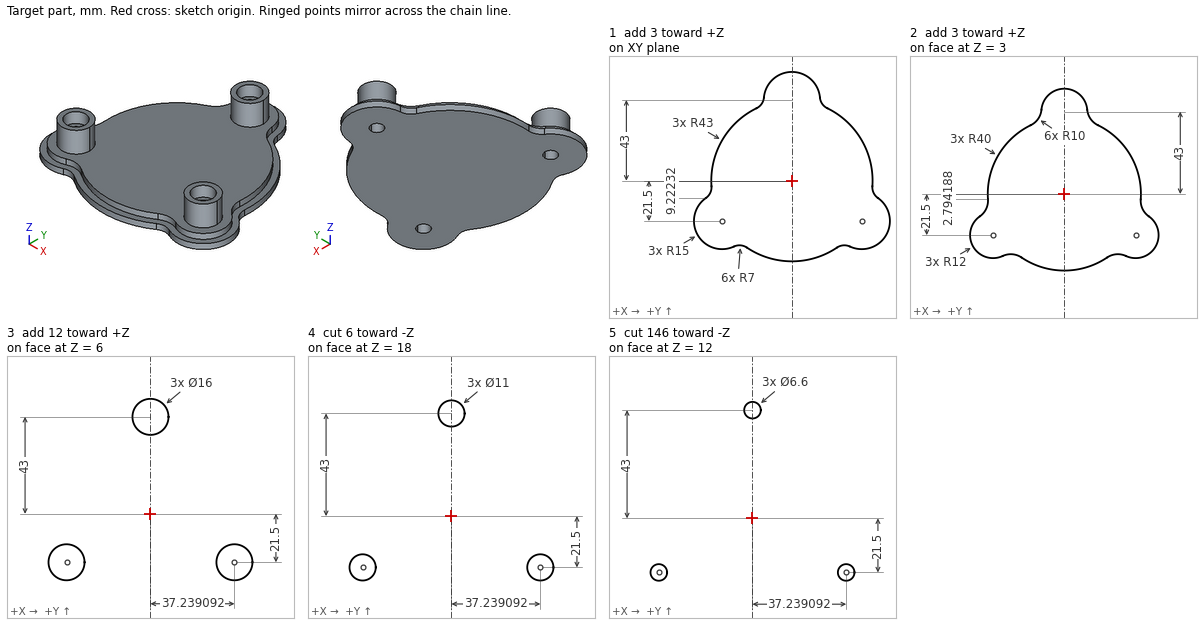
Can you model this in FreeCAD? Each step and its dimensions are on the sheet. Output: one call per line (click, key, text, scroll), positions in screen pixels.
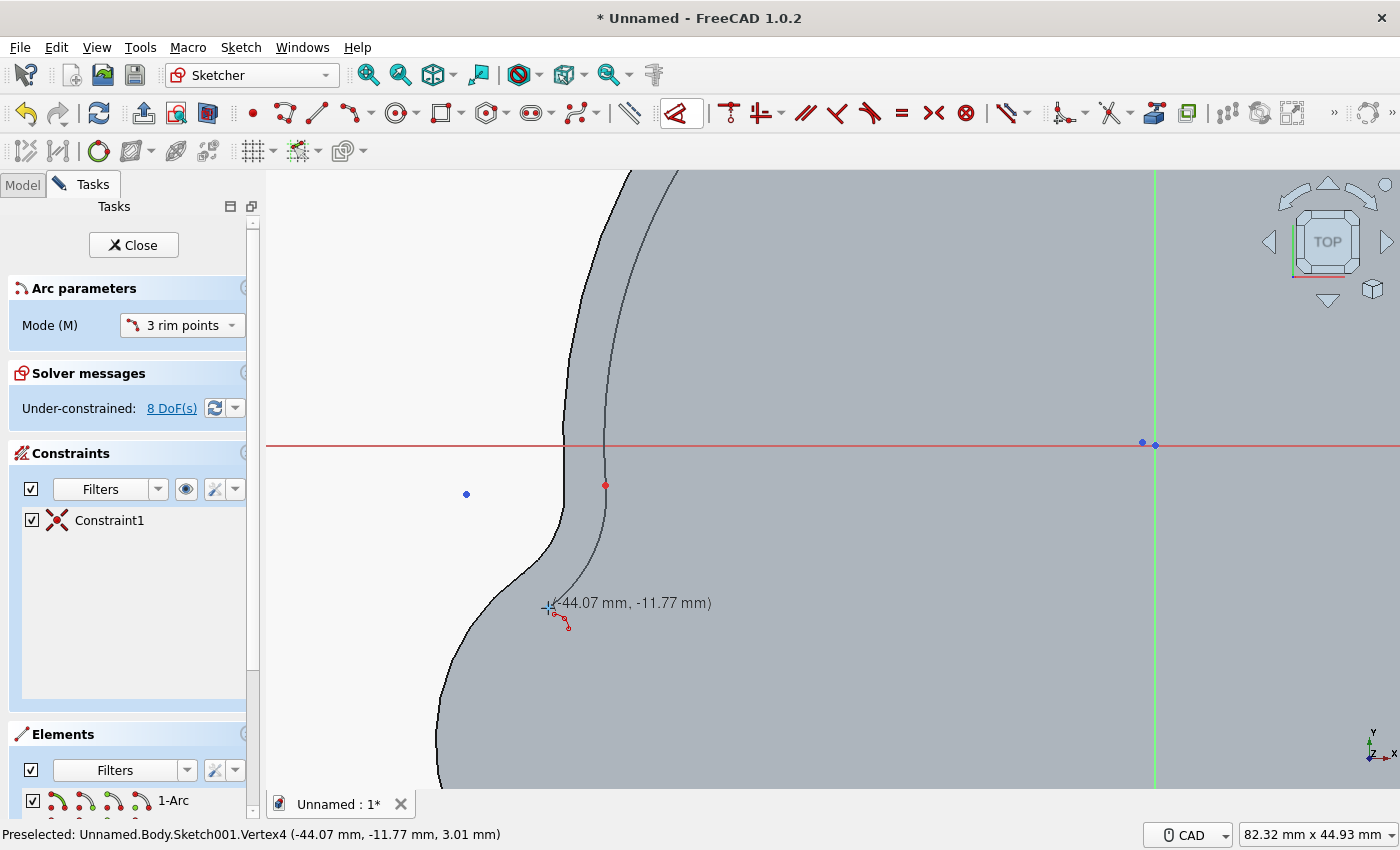
scroll(596, 539, down, 6)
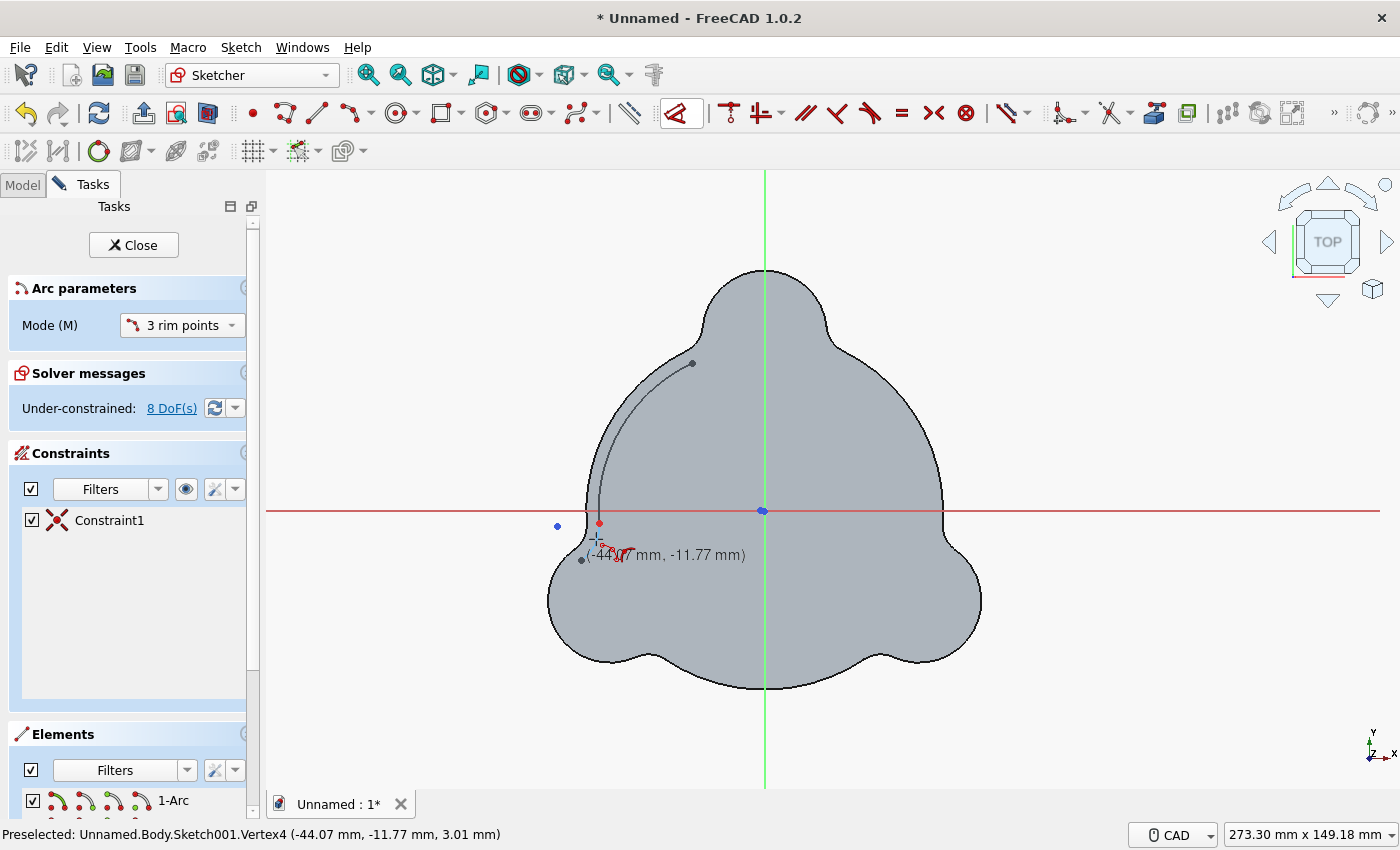
click(631, 646)
click(567, 625)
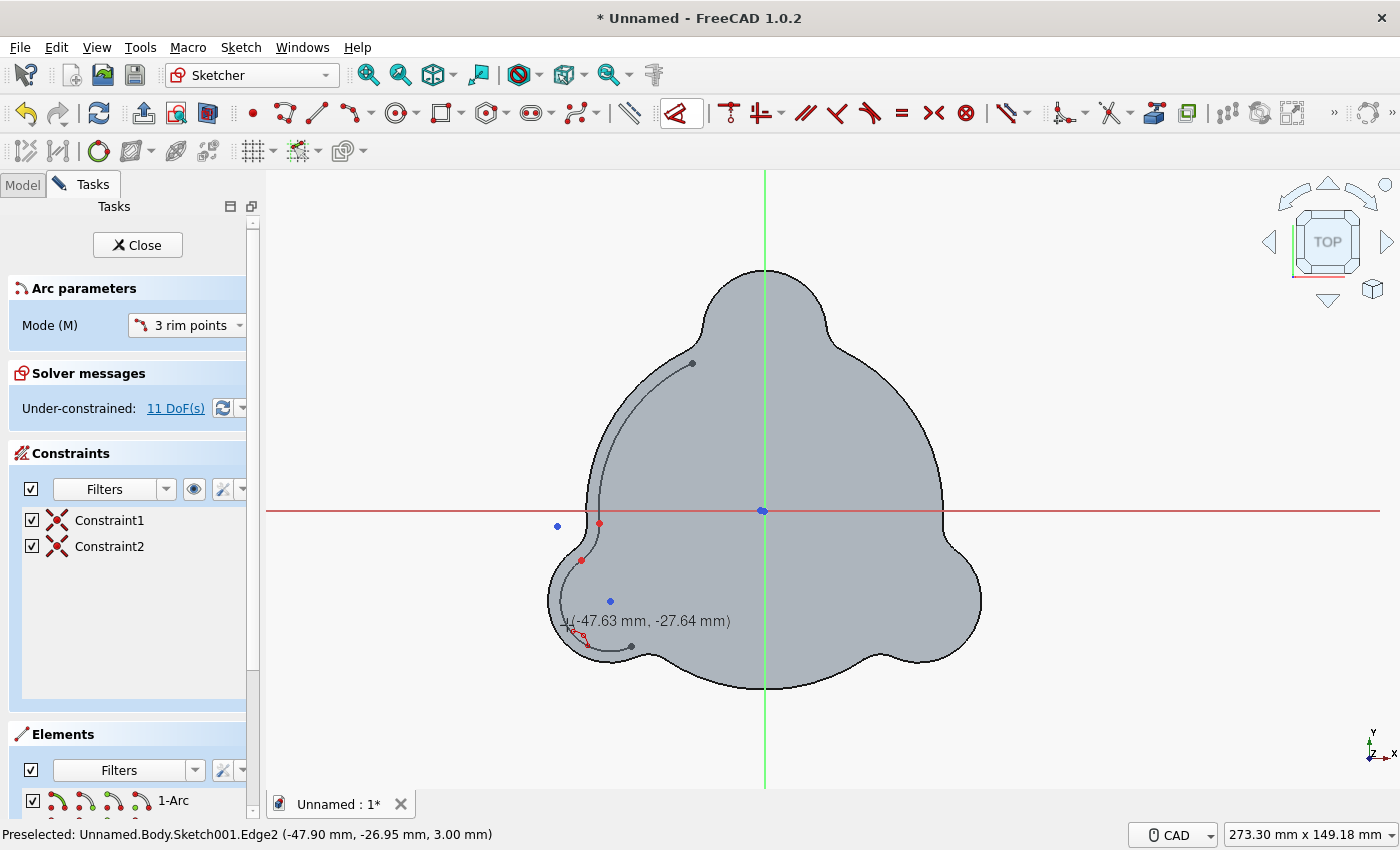
click(631, 647)
click(672, 649)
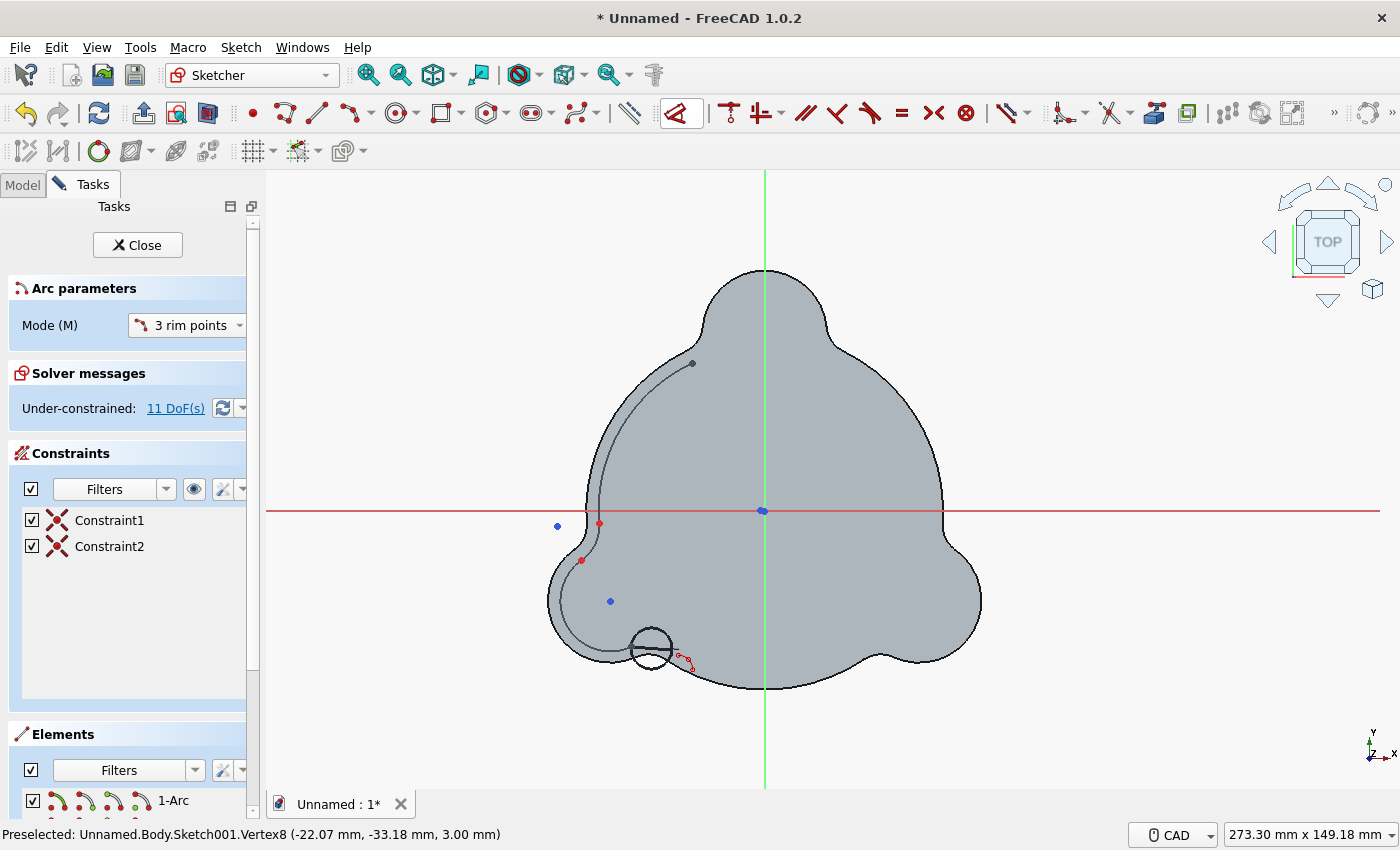
scroll(652, 642, up, 6)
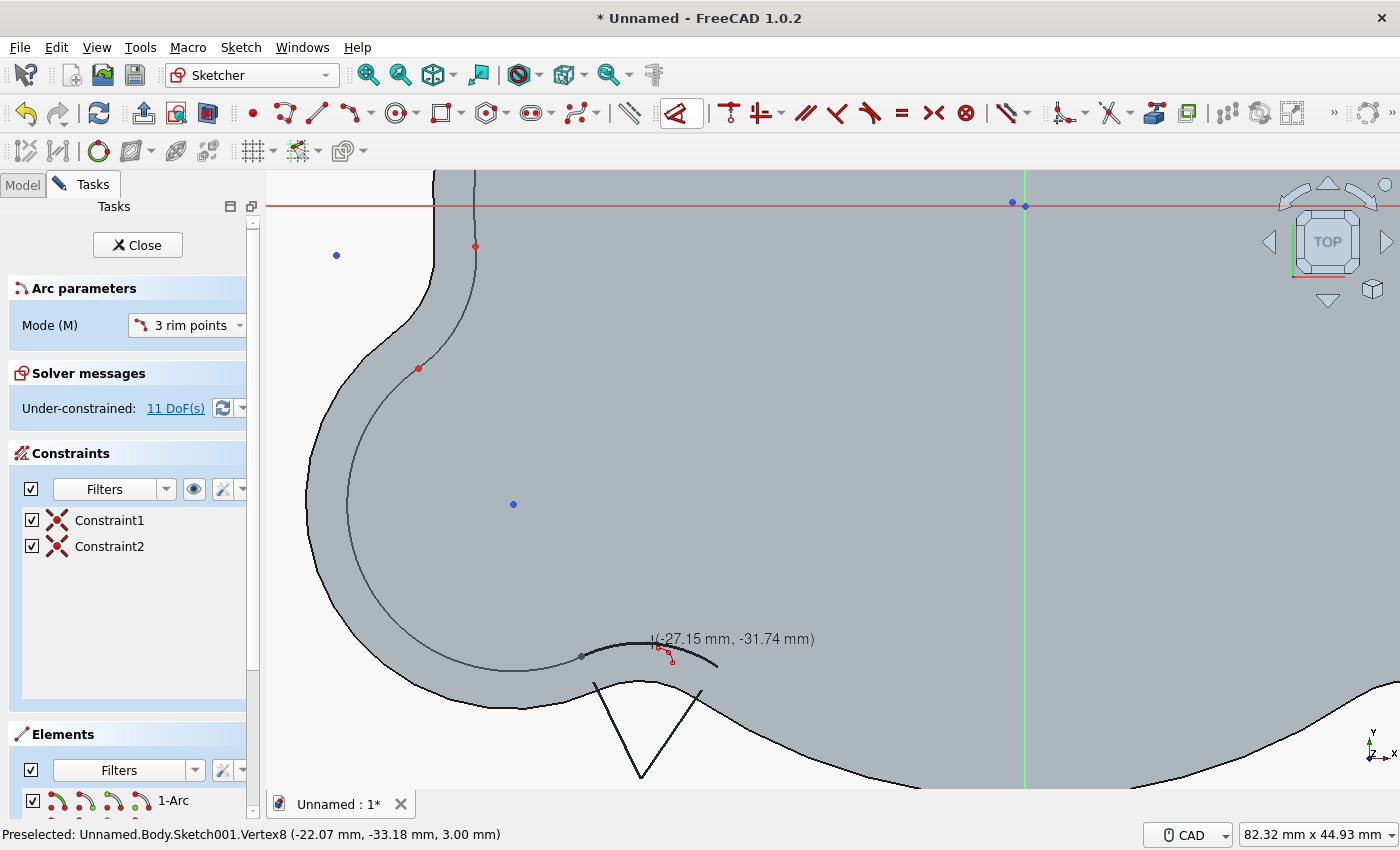
click(651, 640)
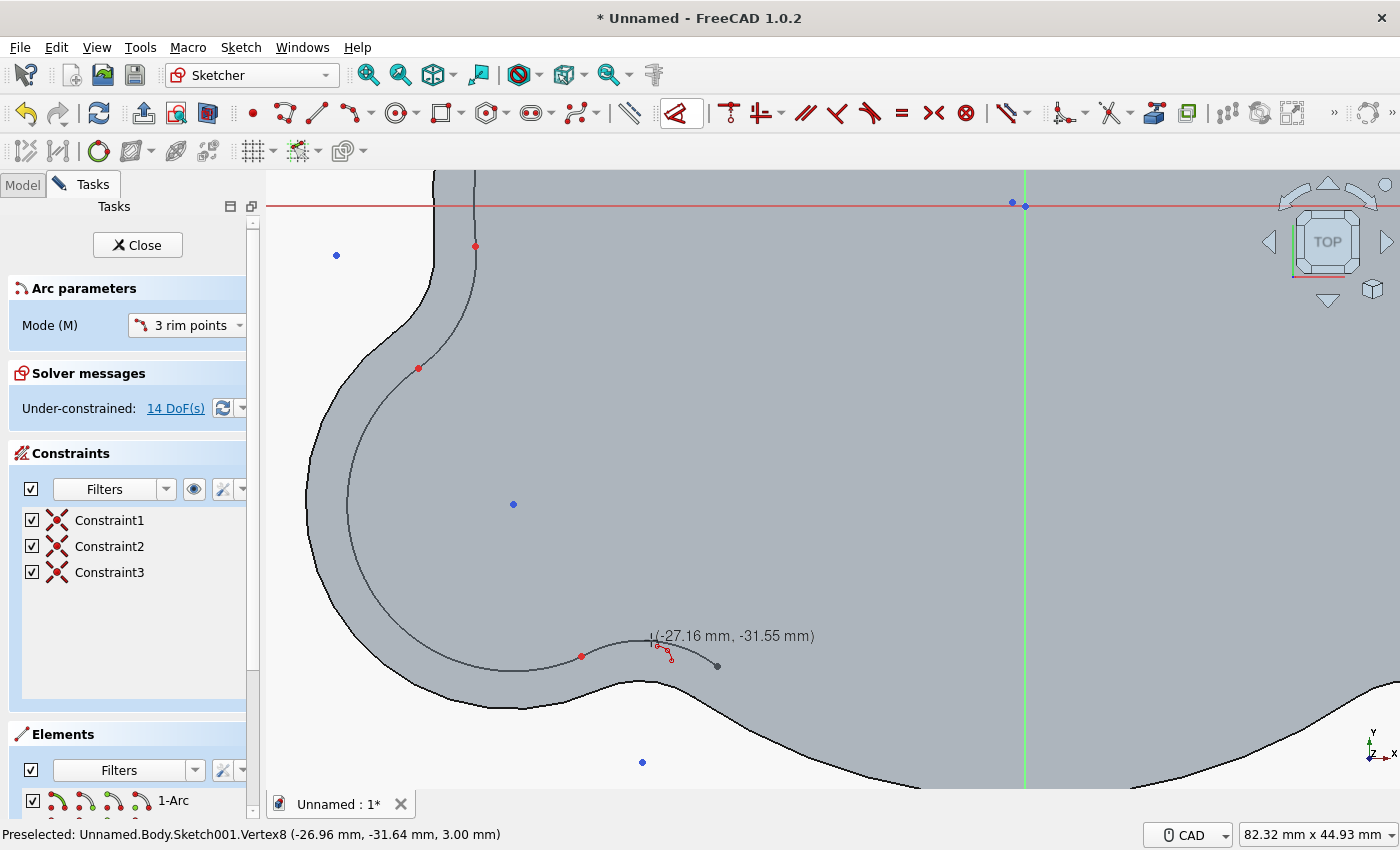
click(718, 667)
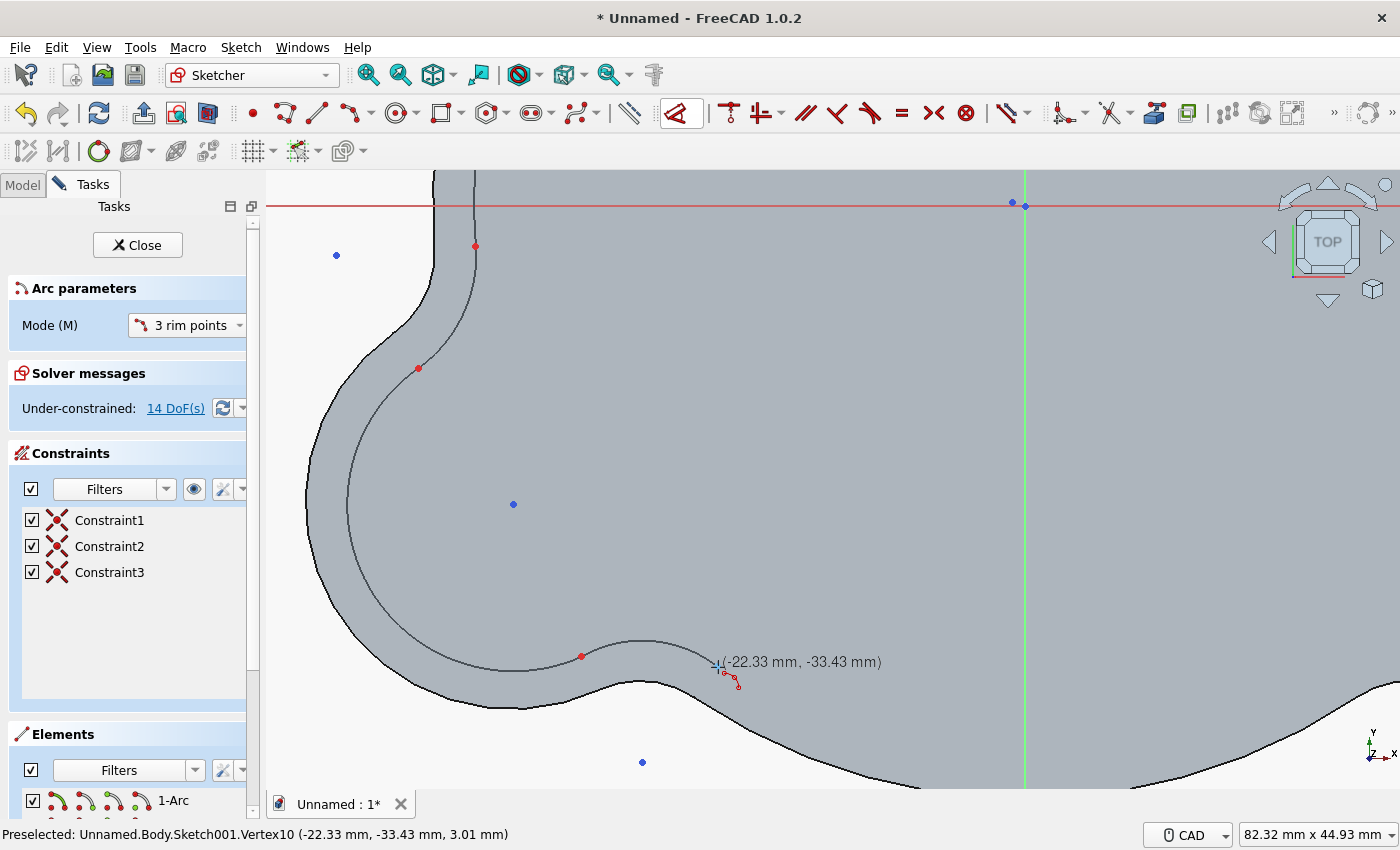
scroll(652, 642, down, 6)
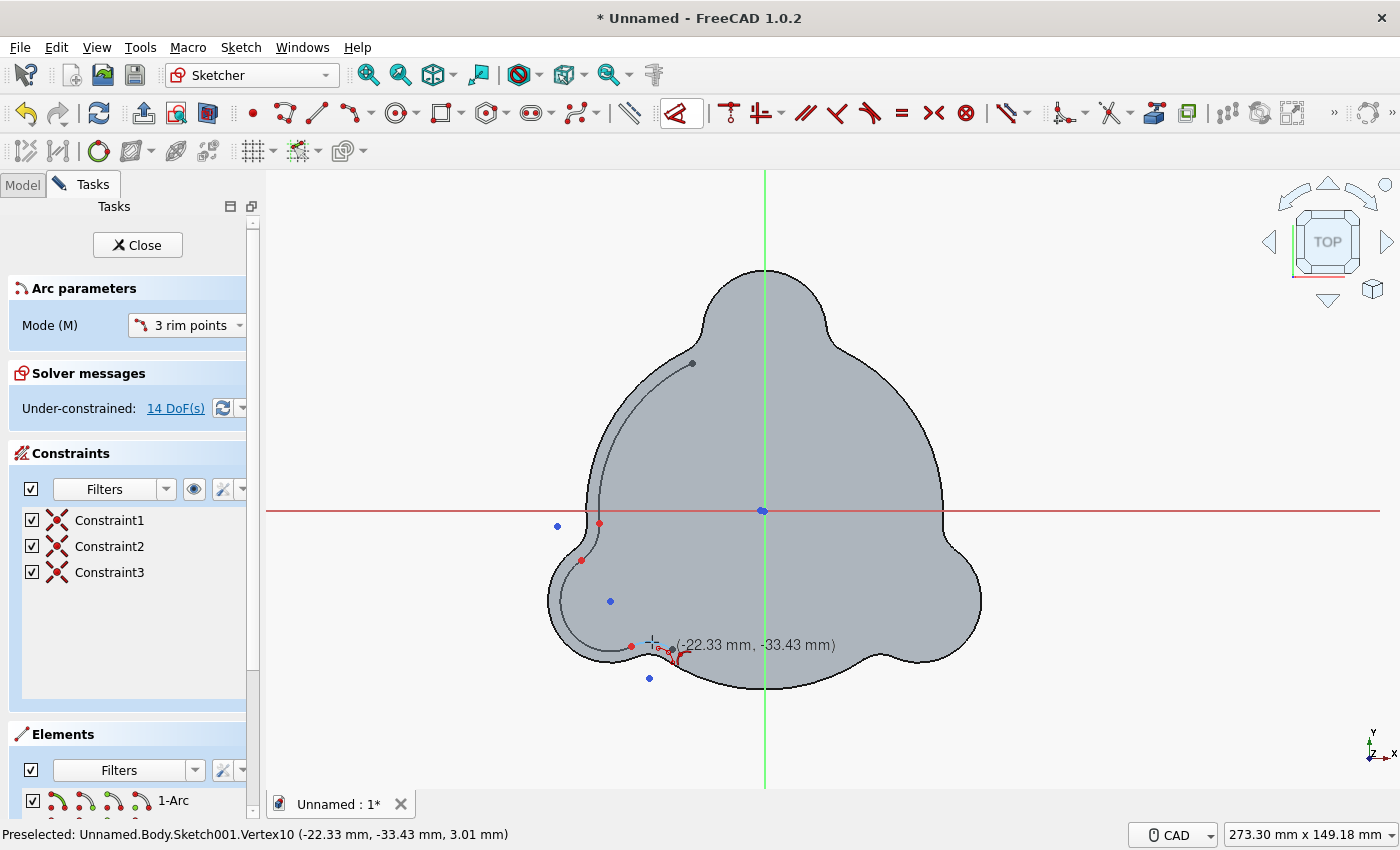
click(857, 649)
click(745, 676)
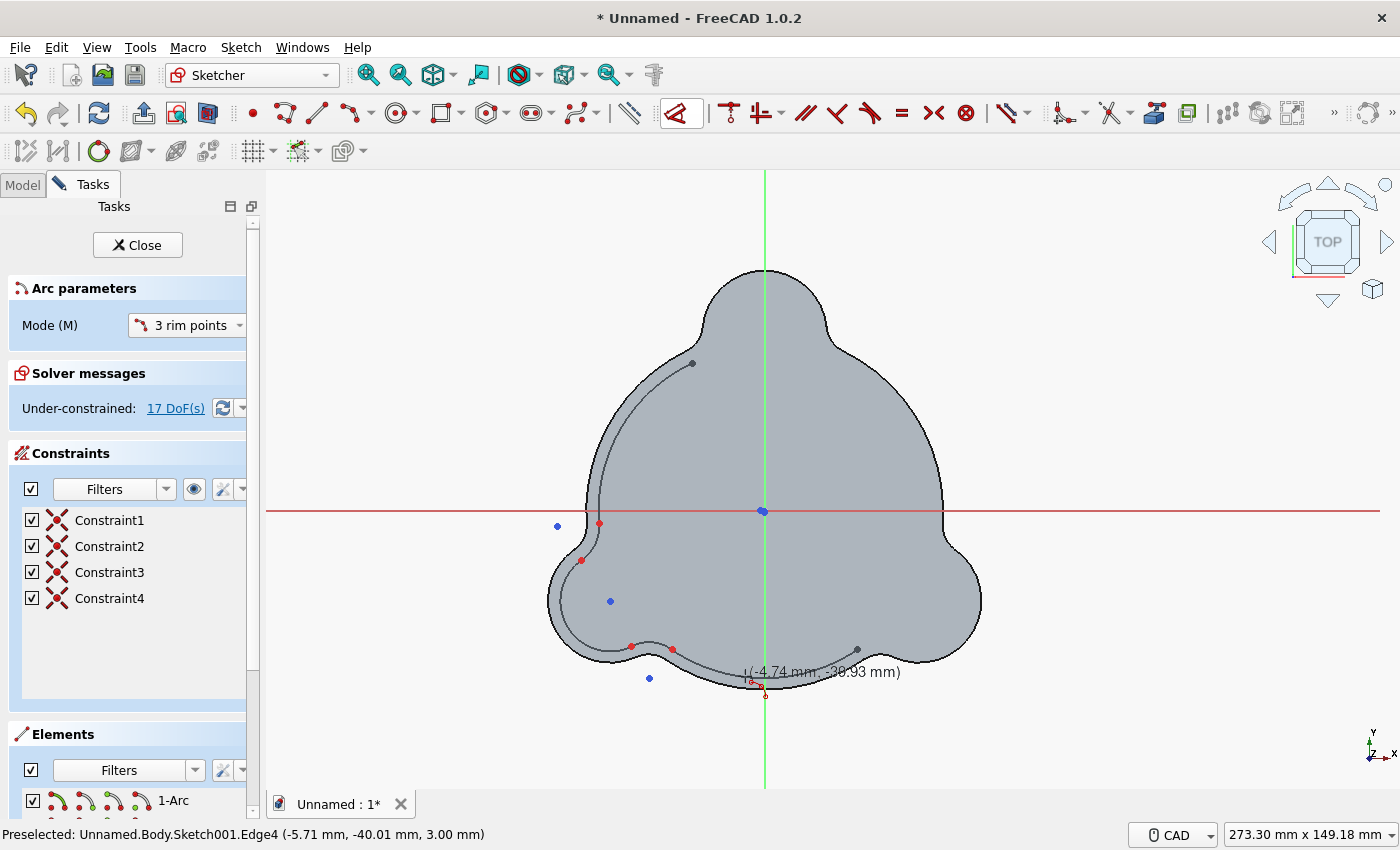
click(857, 650)
click(898, 646)